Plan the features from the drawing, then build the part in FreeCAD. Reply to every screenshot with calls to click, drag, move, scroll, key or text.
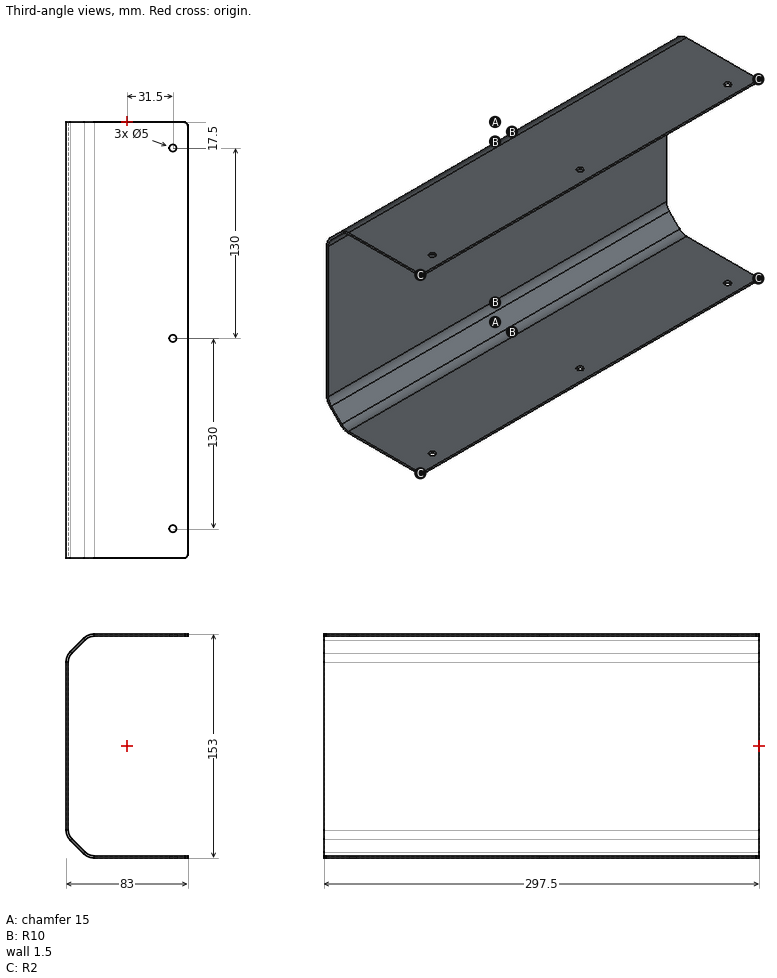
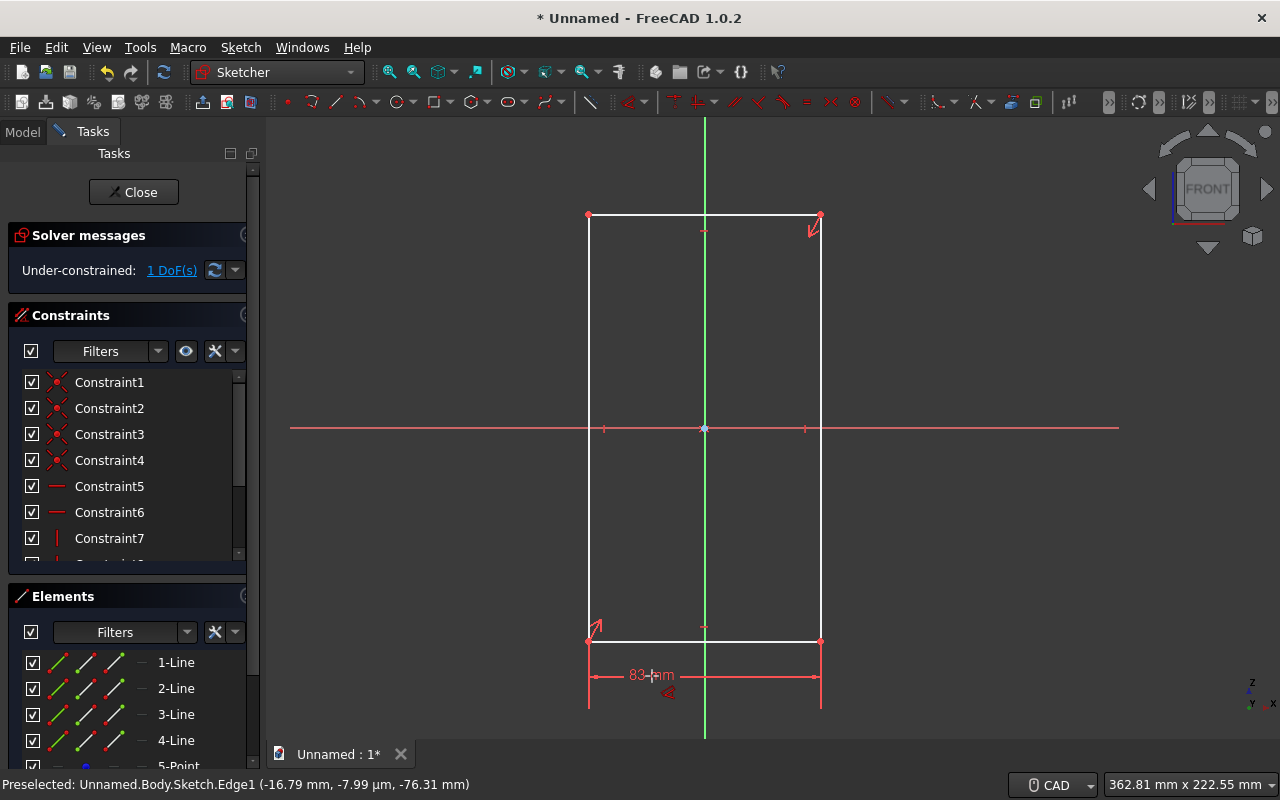
click(821, 514)
click(855, 330)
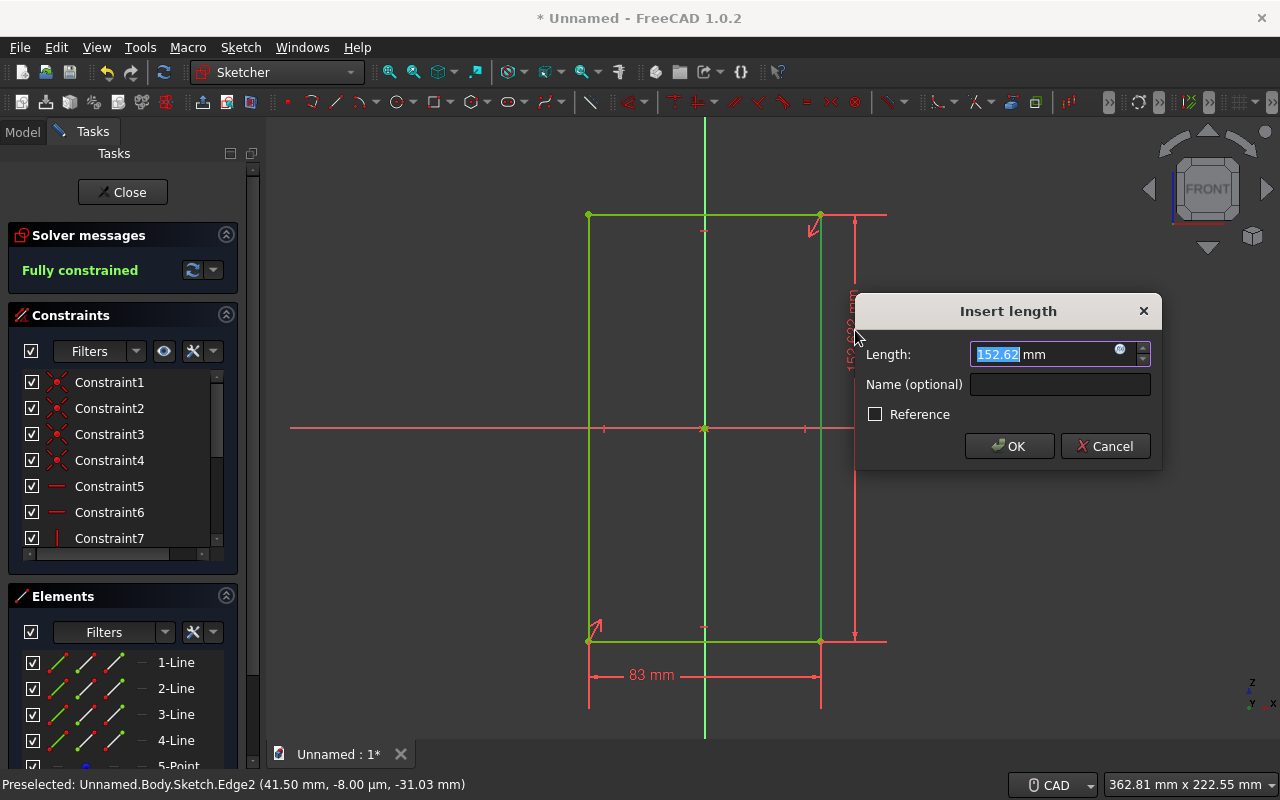
text(153)
key(Return)
key(Escape)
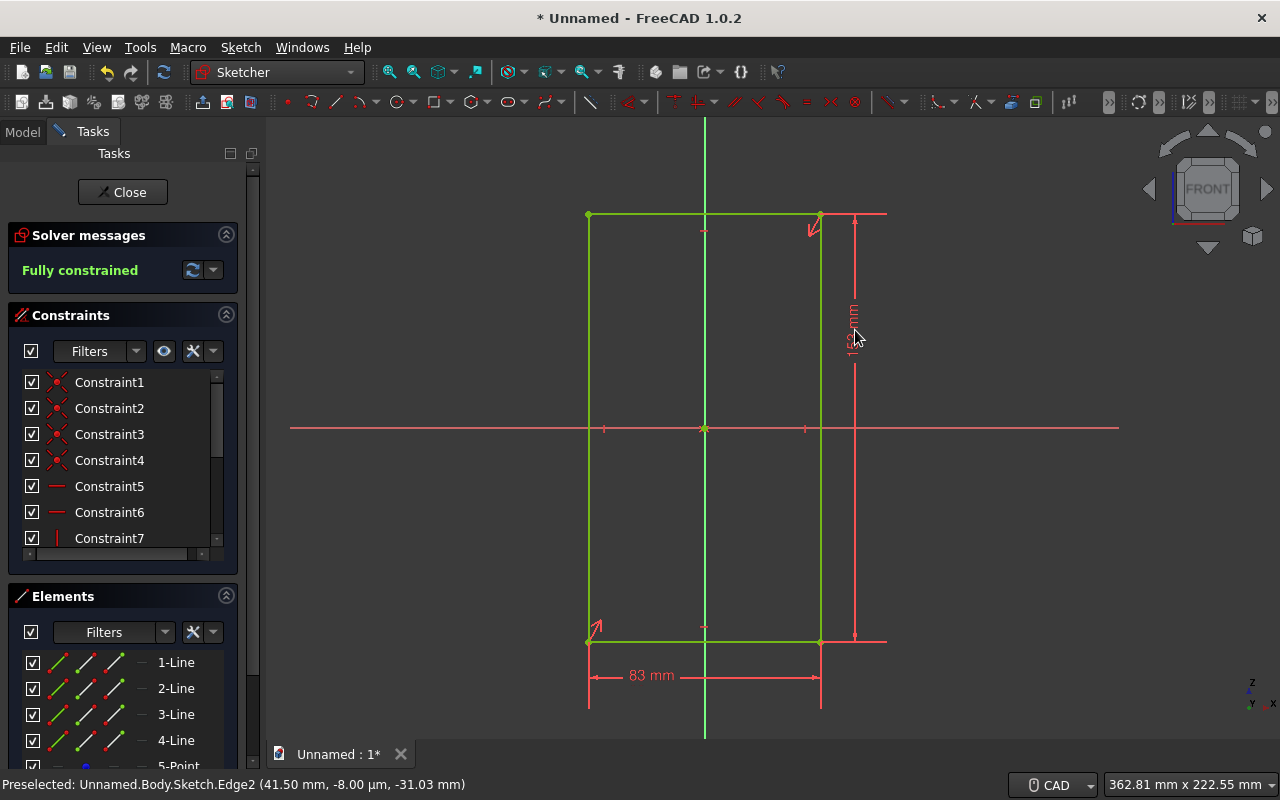
click(123, 192)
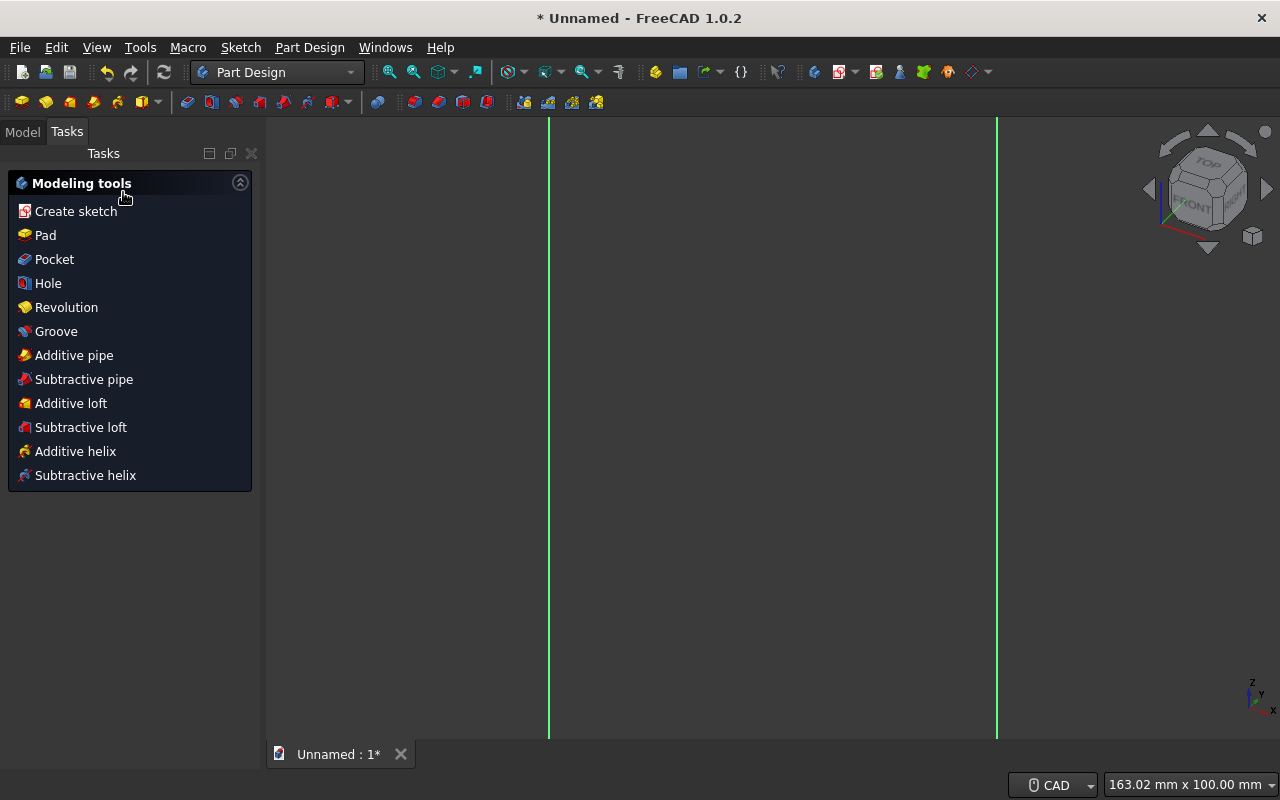
click(22, 102)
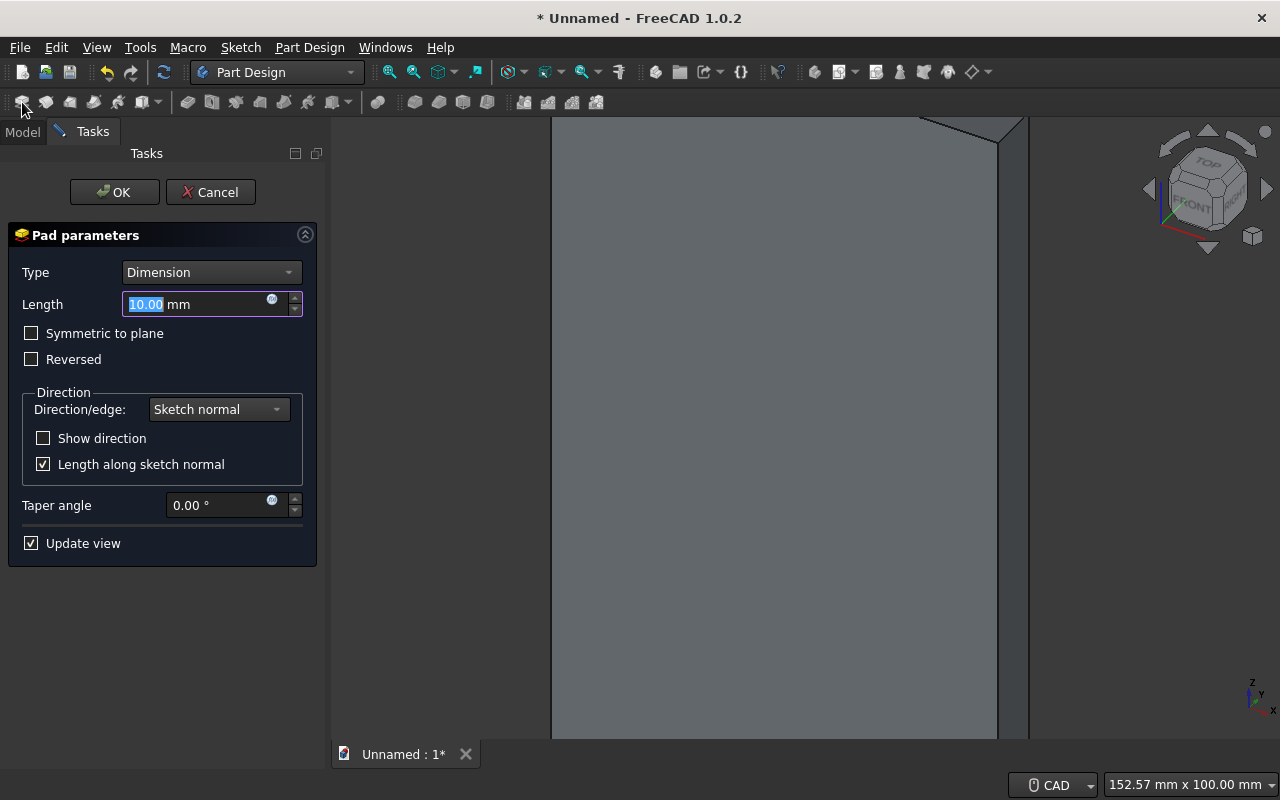
text(297.5)
key(Tab)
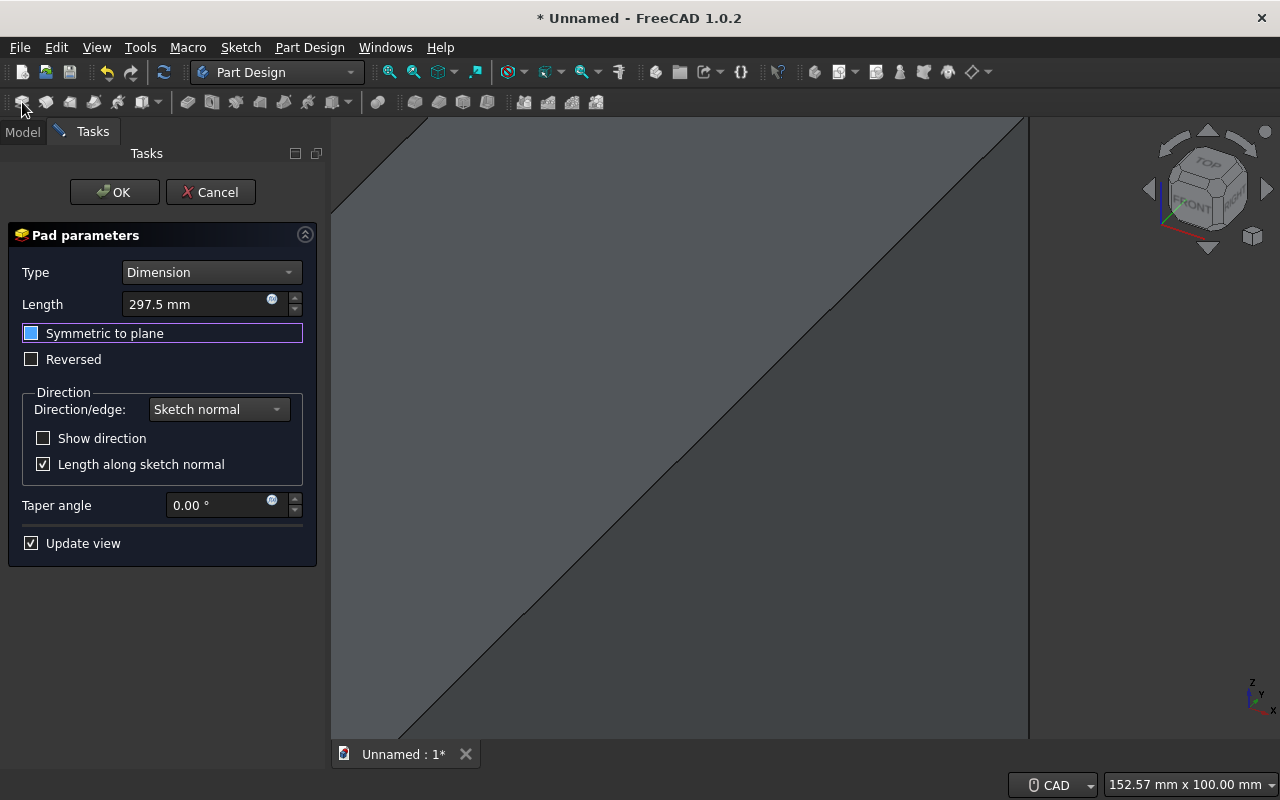
click(115, 192)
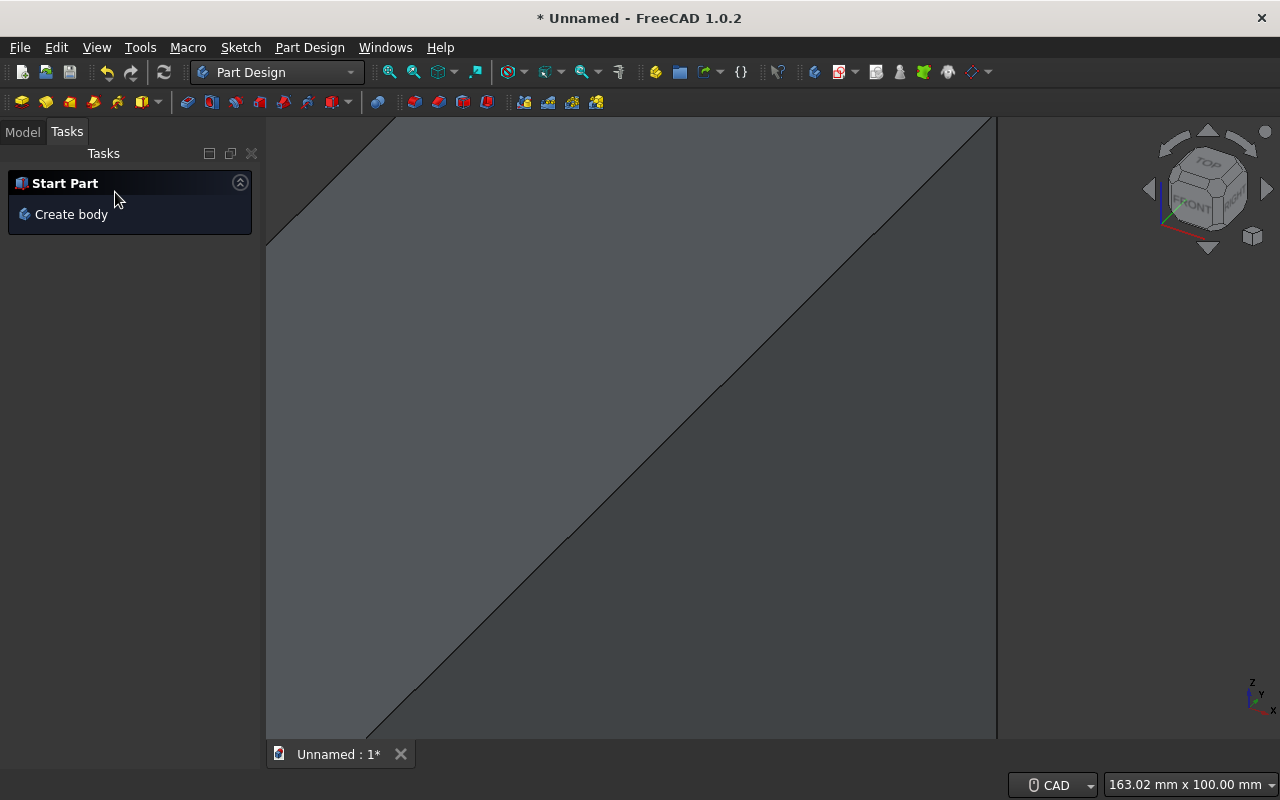
click(390, 72)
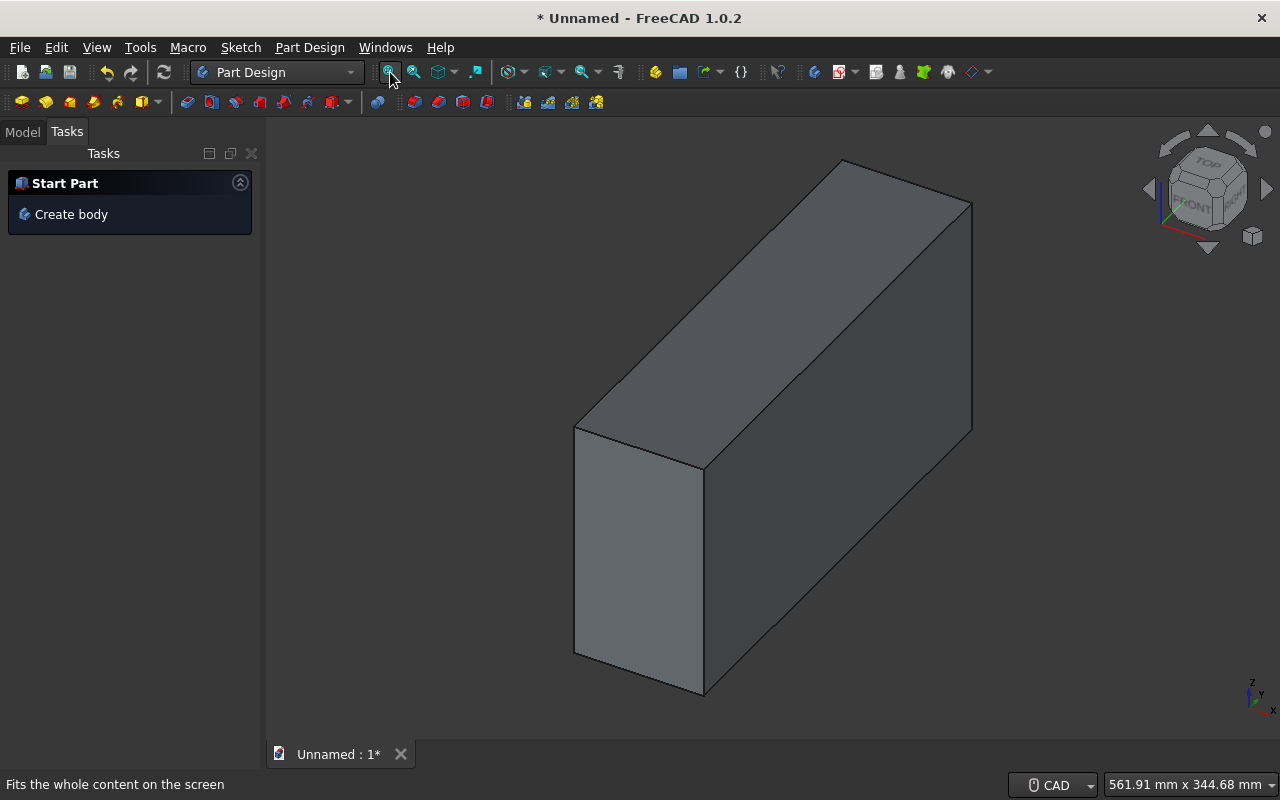
key(0)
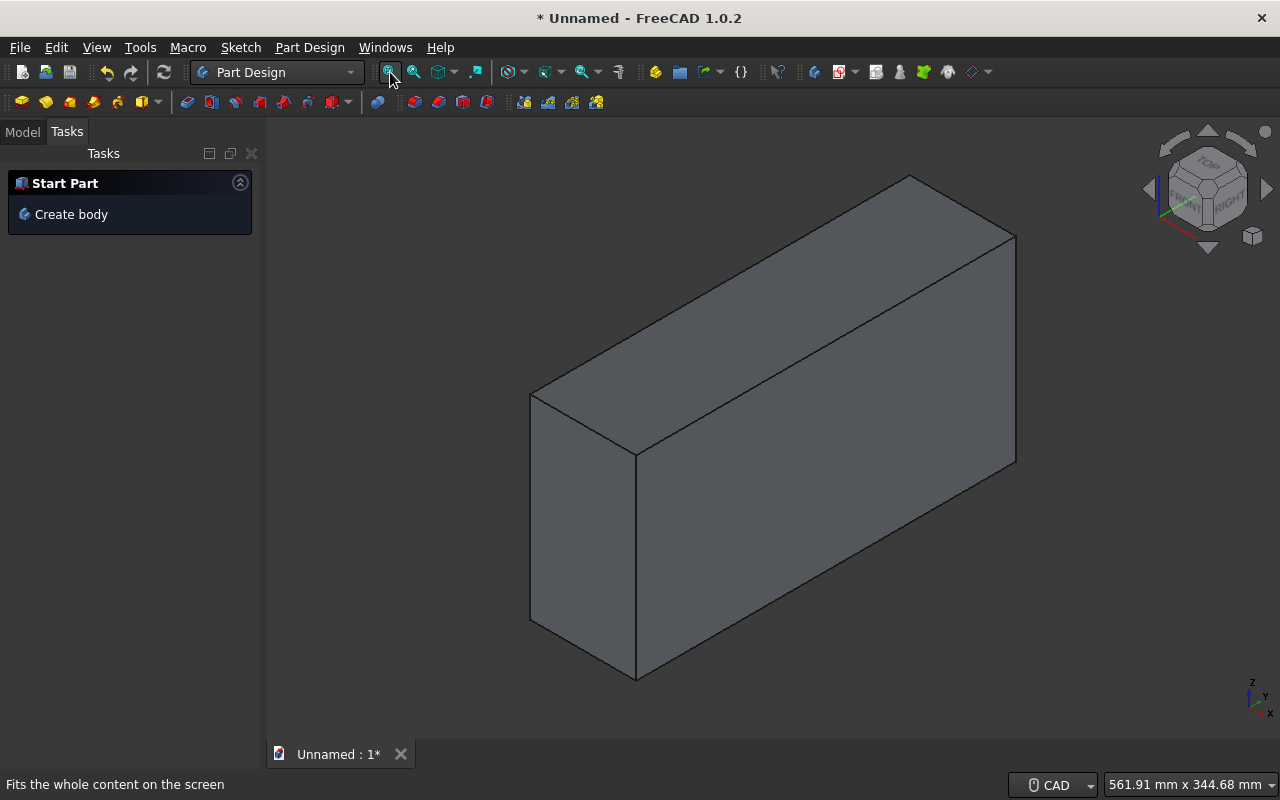
key(2)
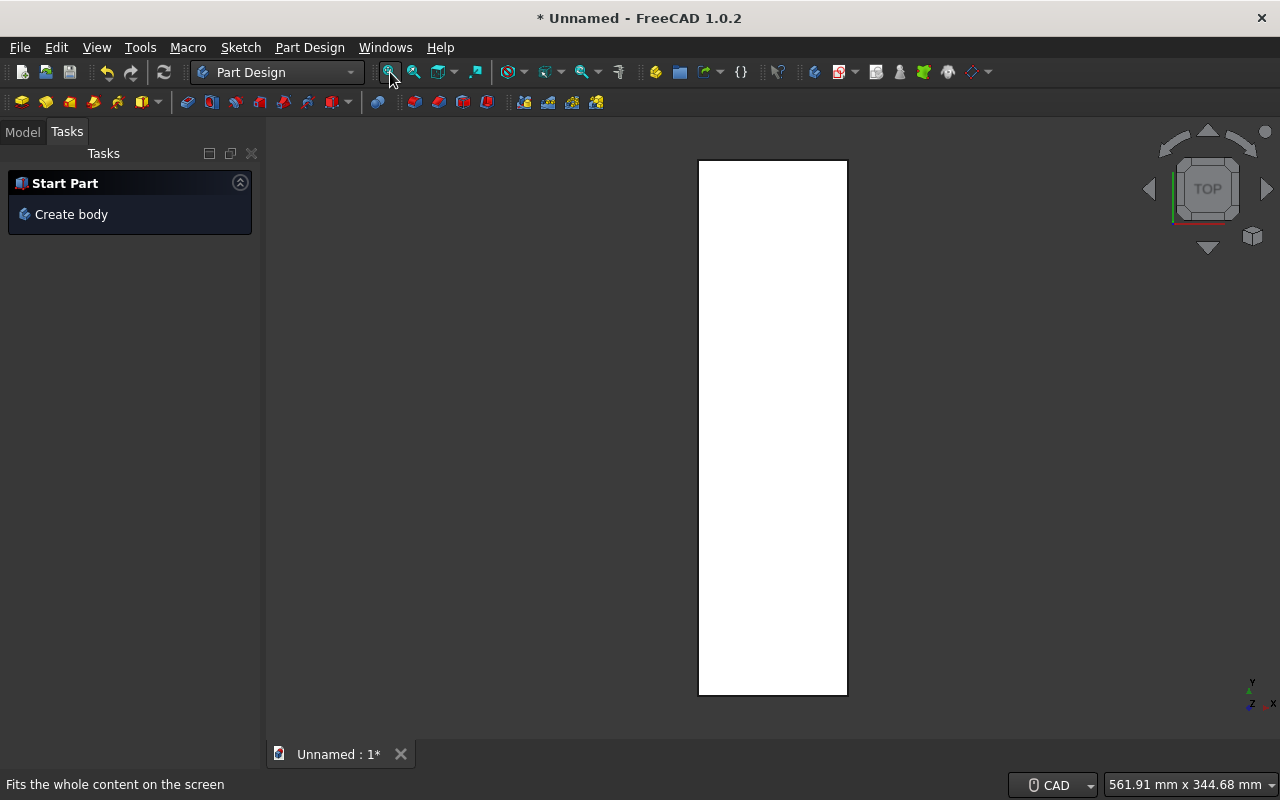
click(698, 427)